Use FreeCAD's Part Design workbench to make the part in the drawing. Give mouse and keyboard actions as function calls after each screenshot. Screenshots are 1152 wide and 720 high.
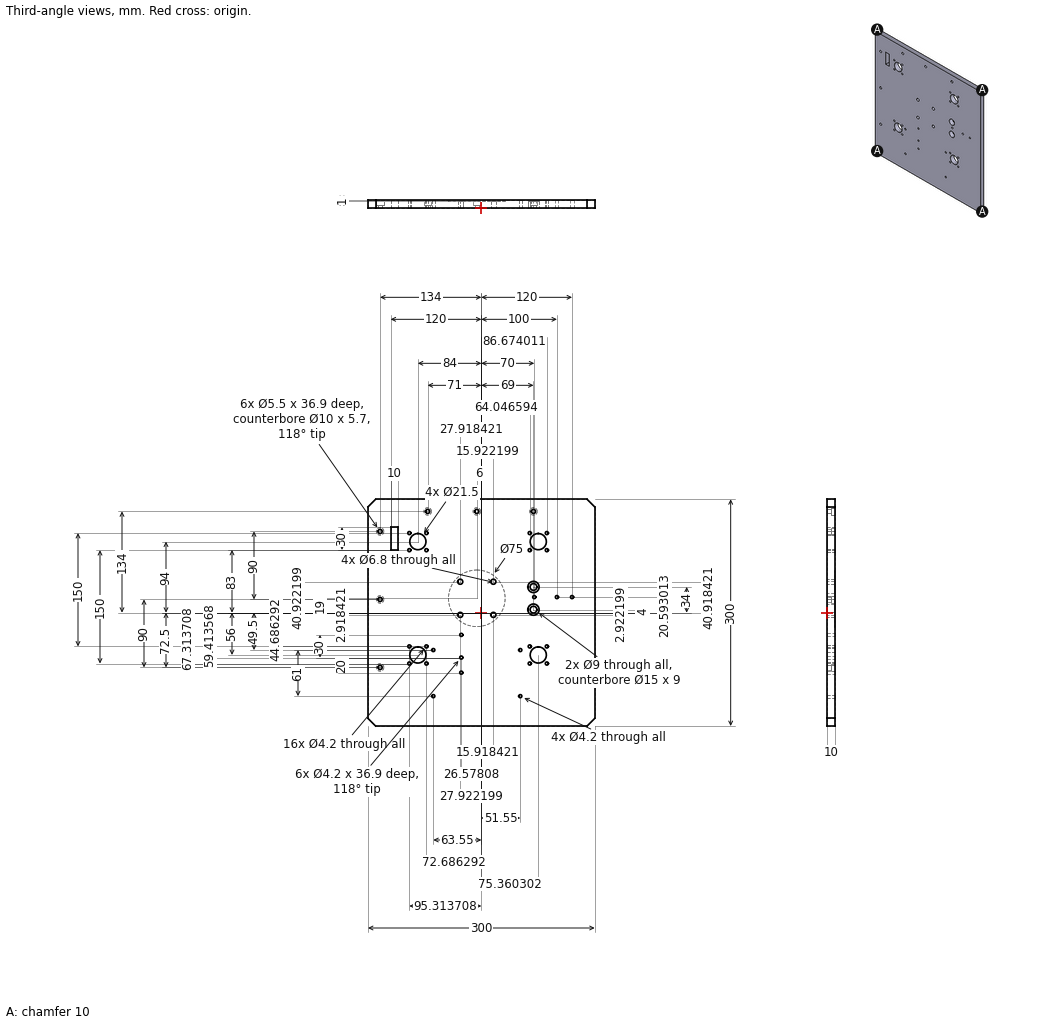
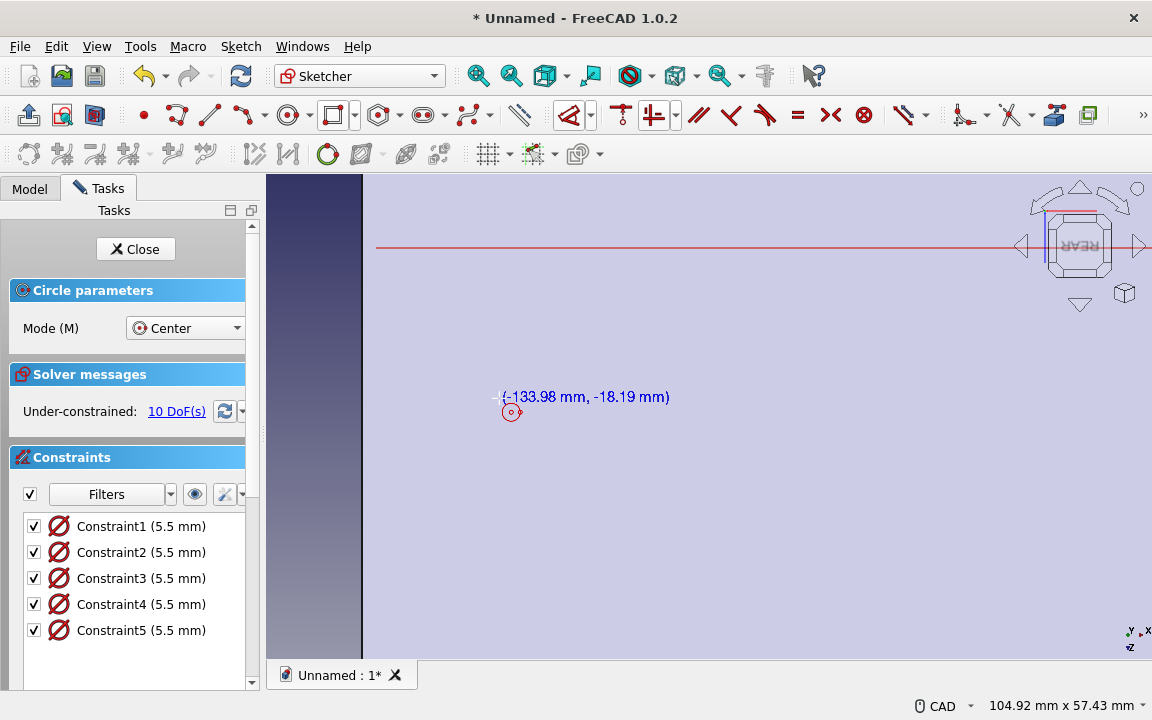
scroll(499, 398, down, 9)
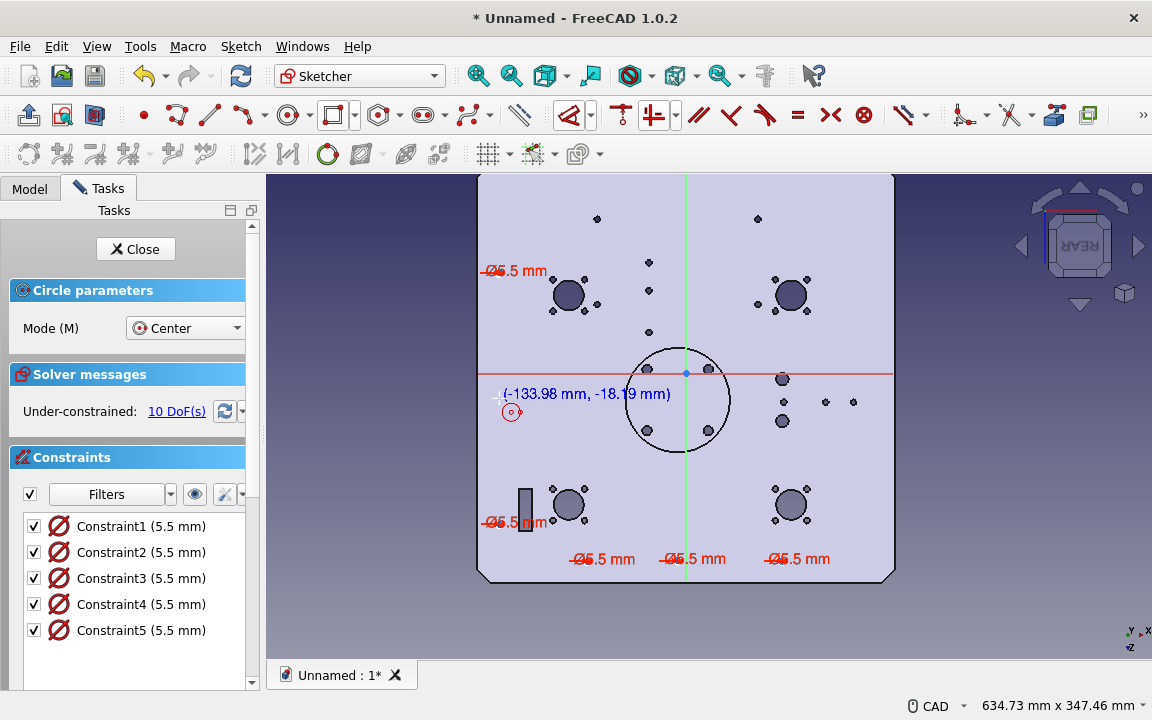
click(499, 398)
move(502, 395)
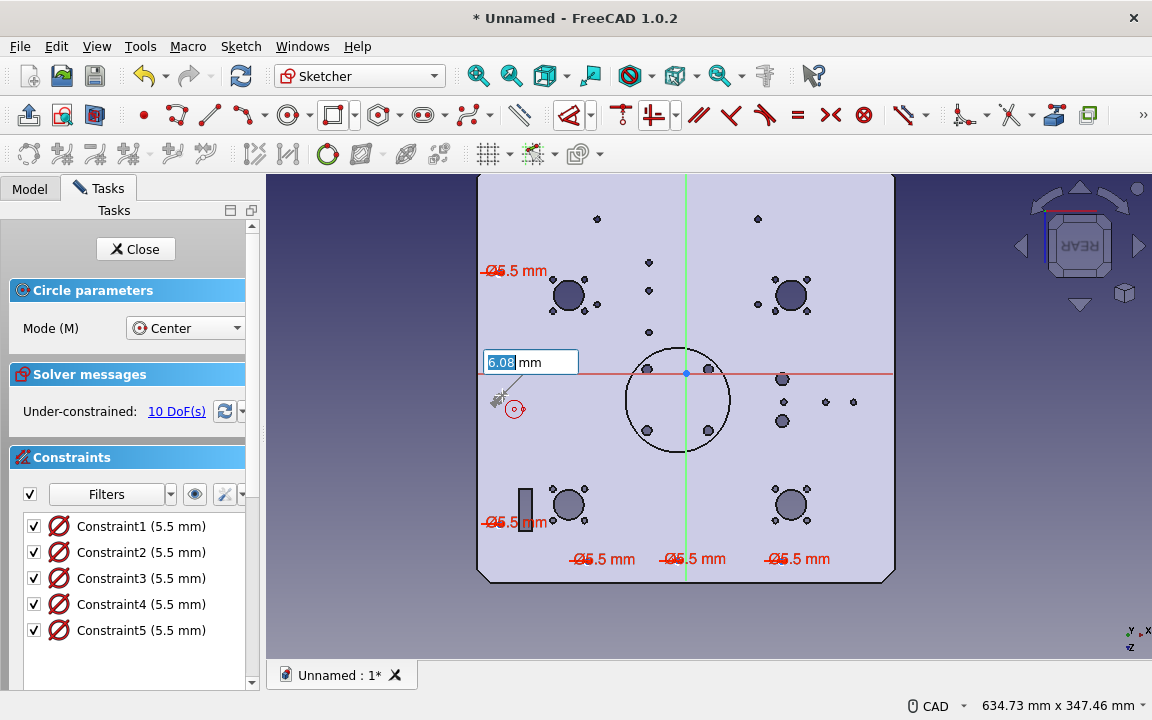
text(5.5)
key(Return)
key(Escape)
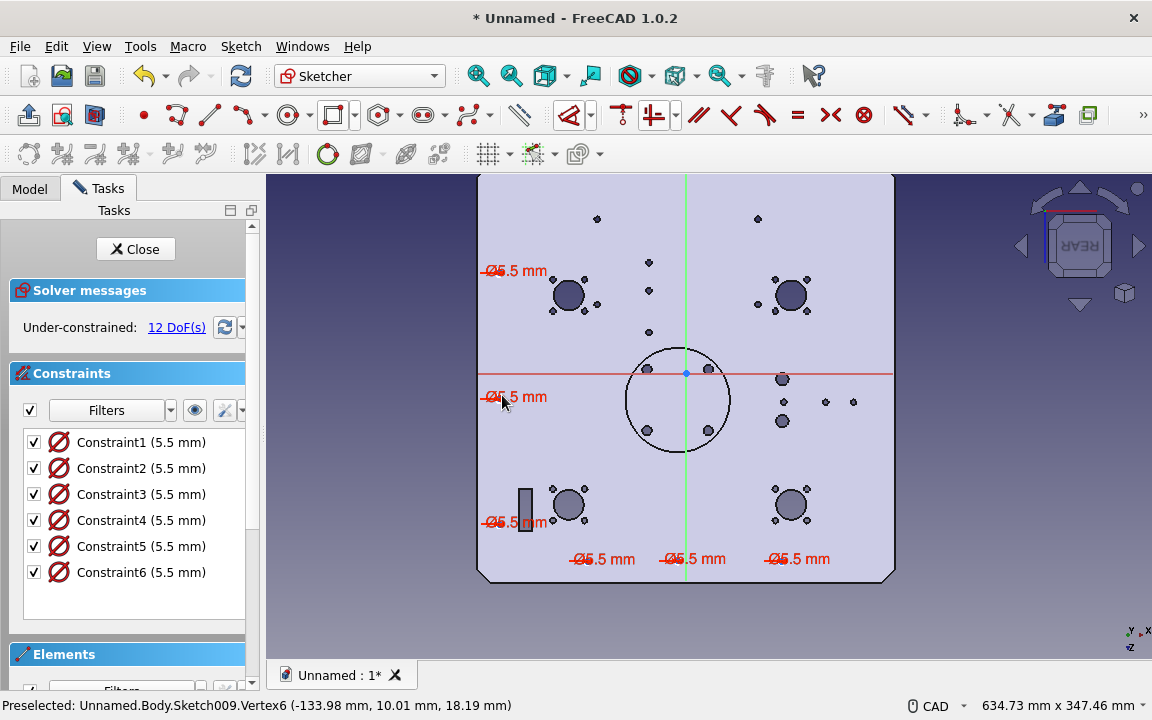
click(587, 561)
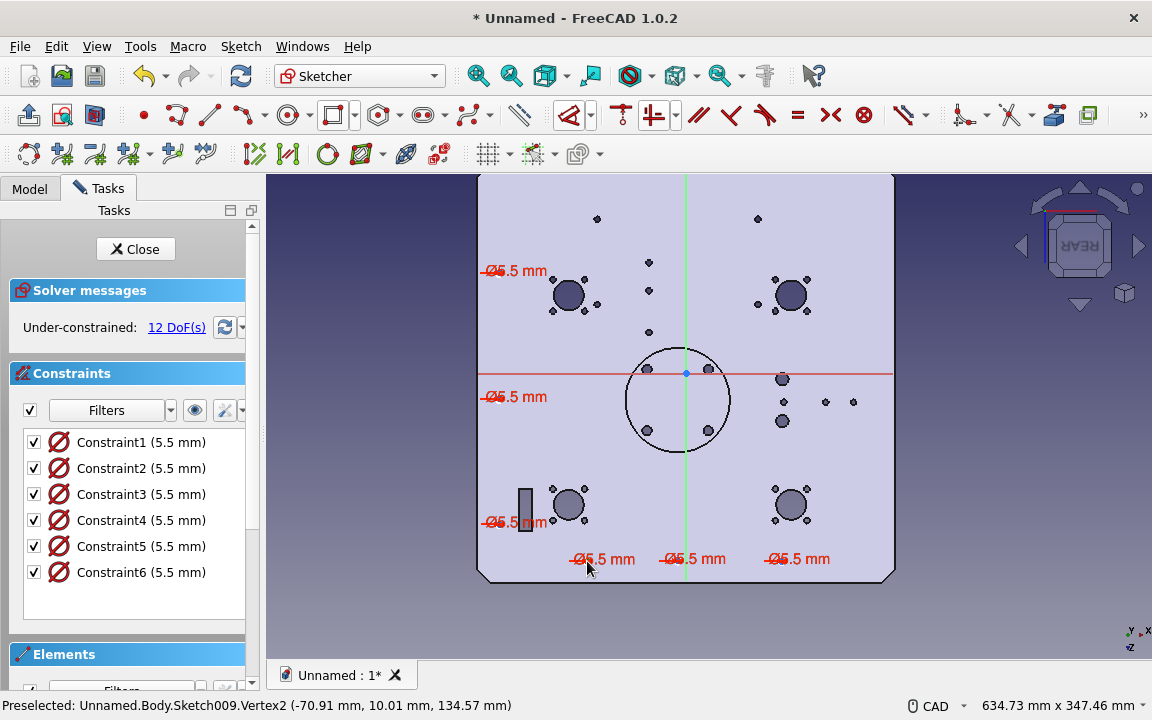
click(678, 561)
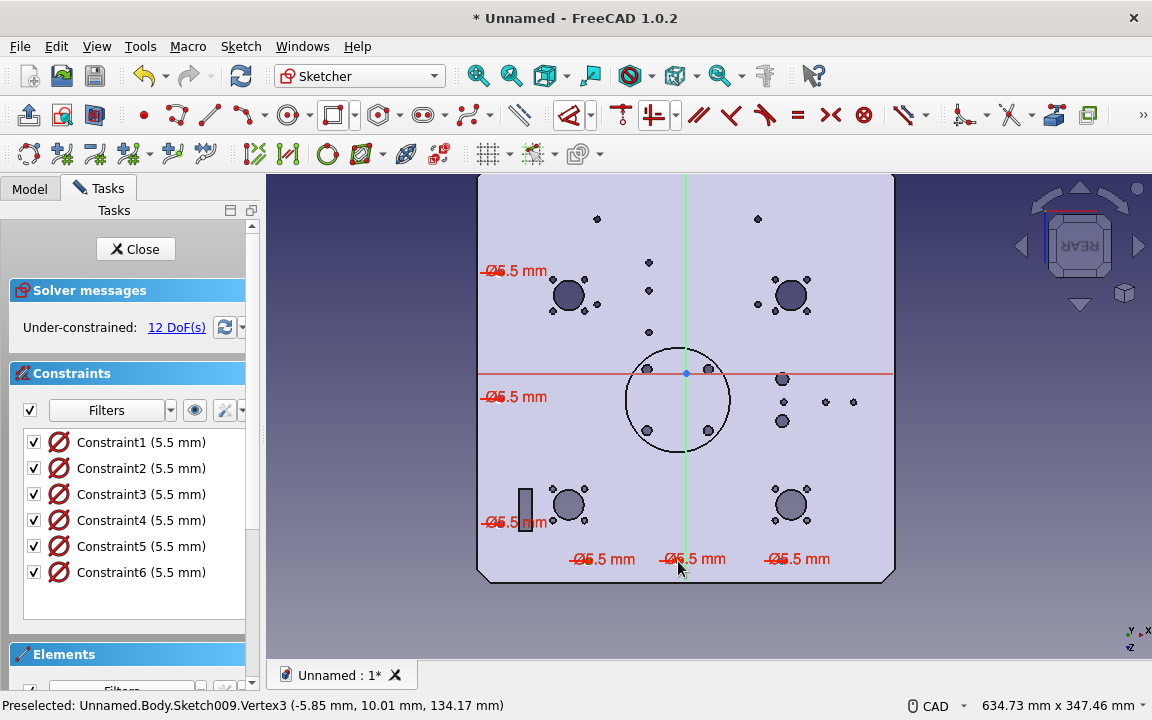
click(676, 116)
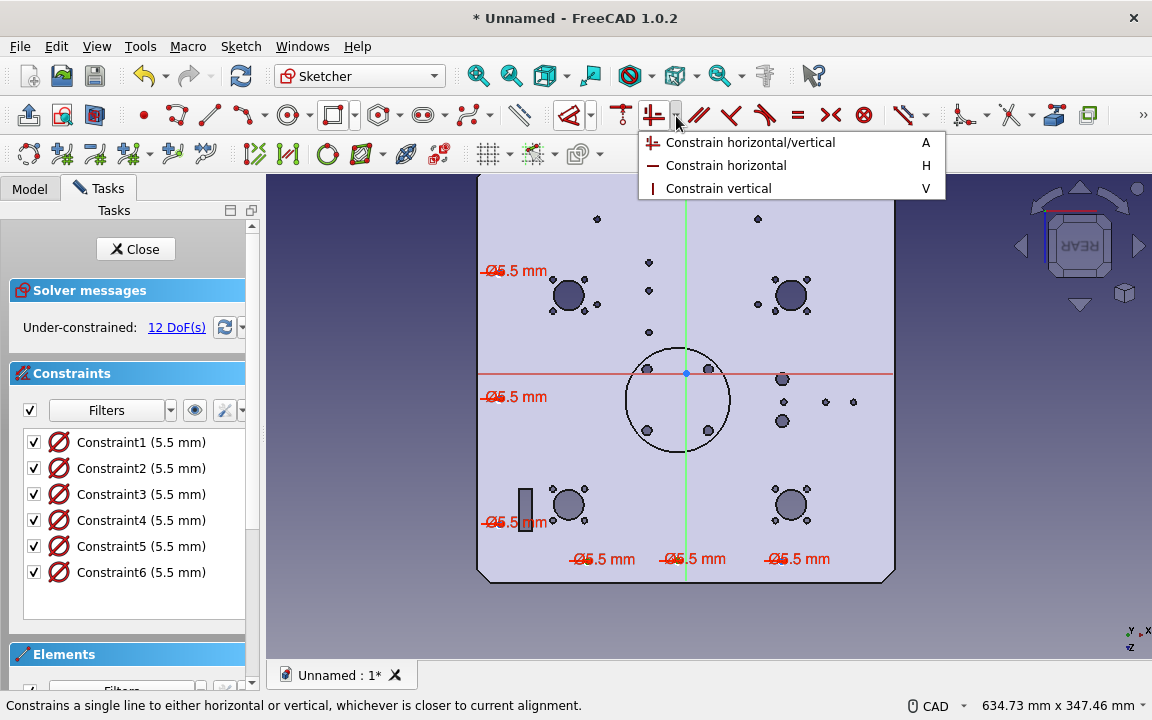
click(792, 166)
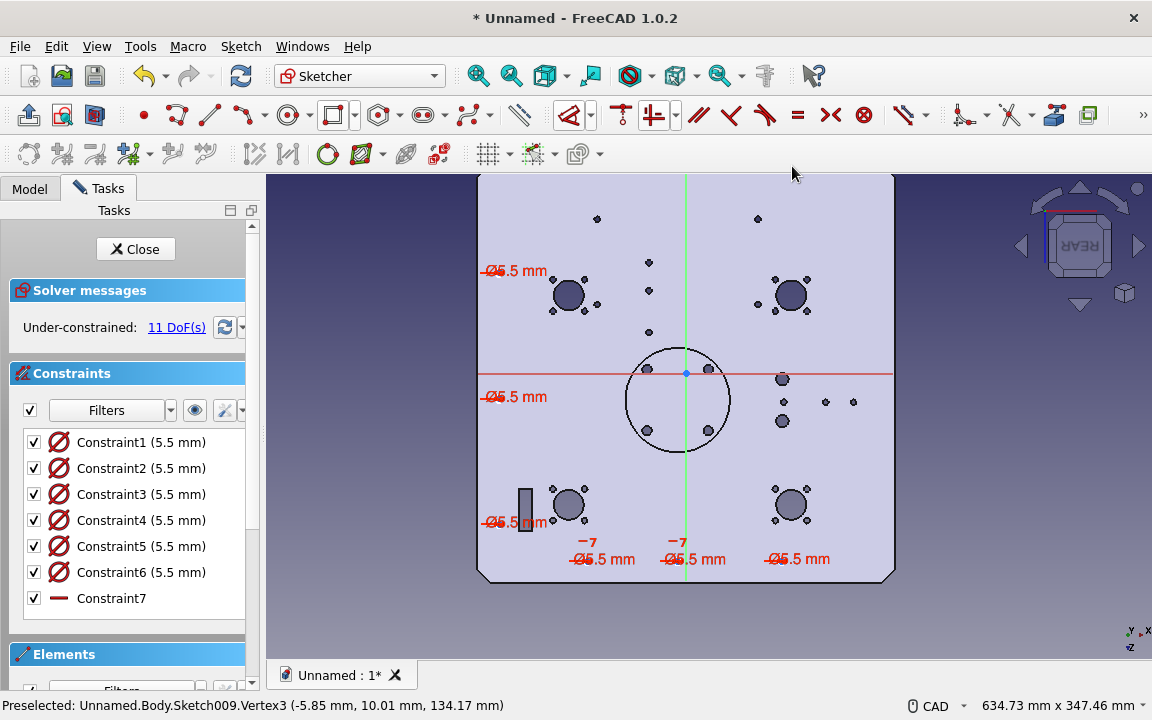
click(678, 561)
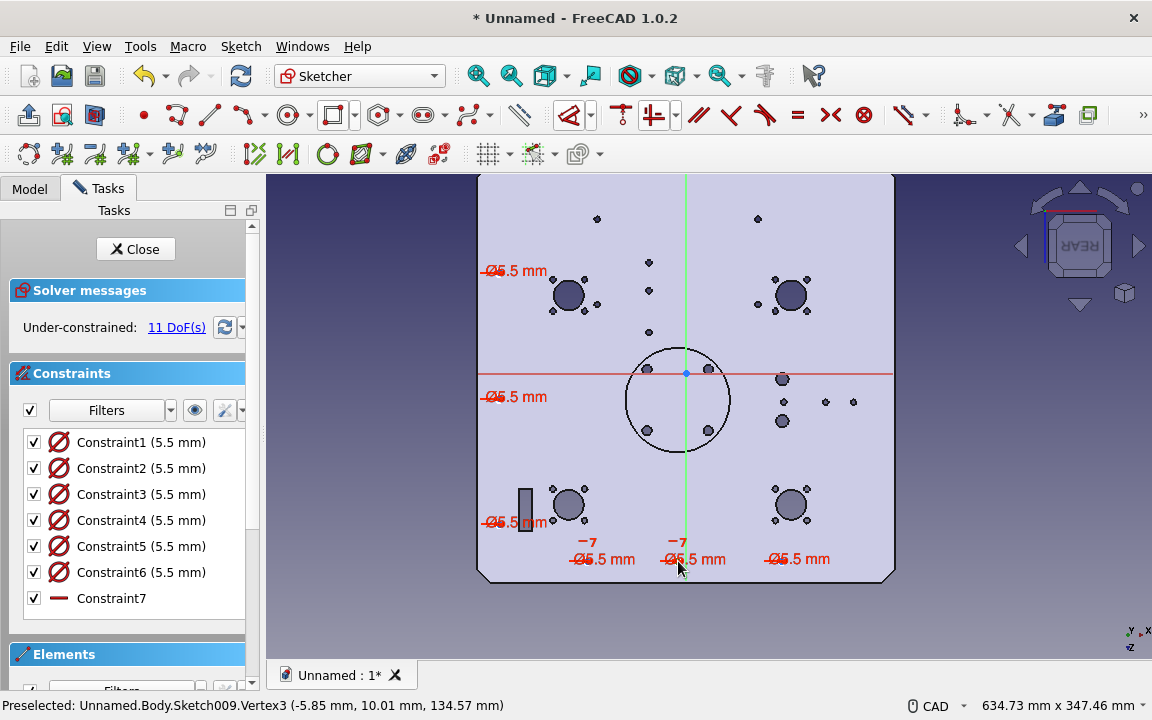
click(782, 561)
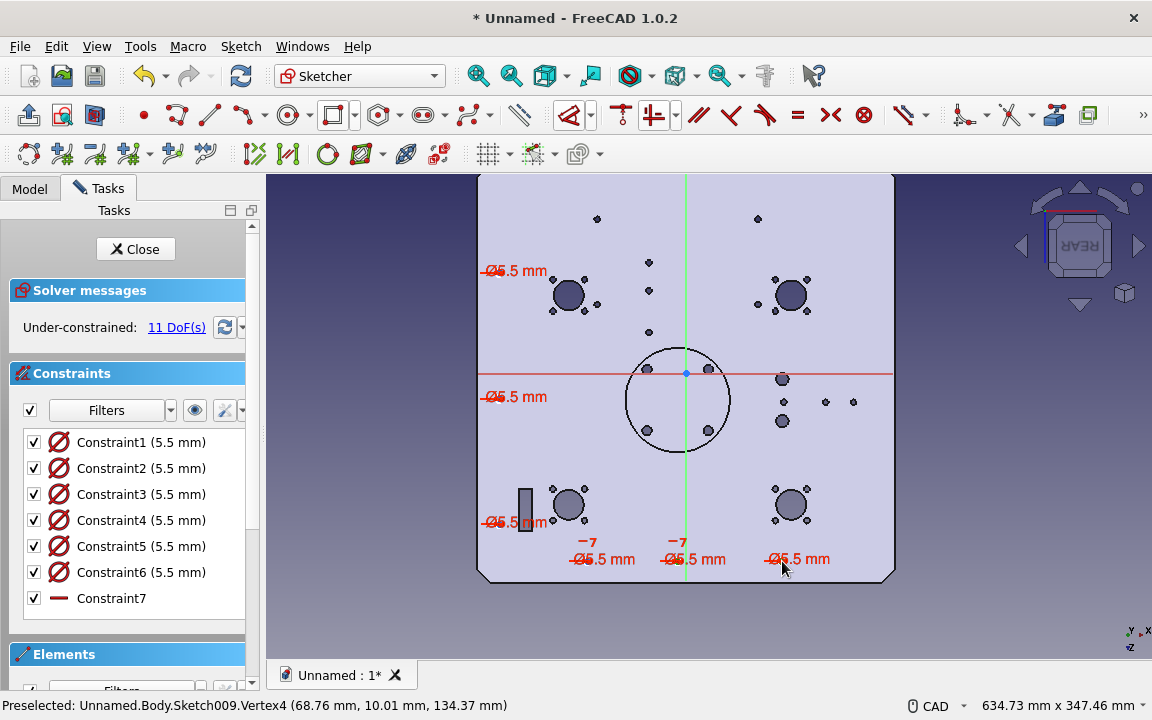
click(676, 116)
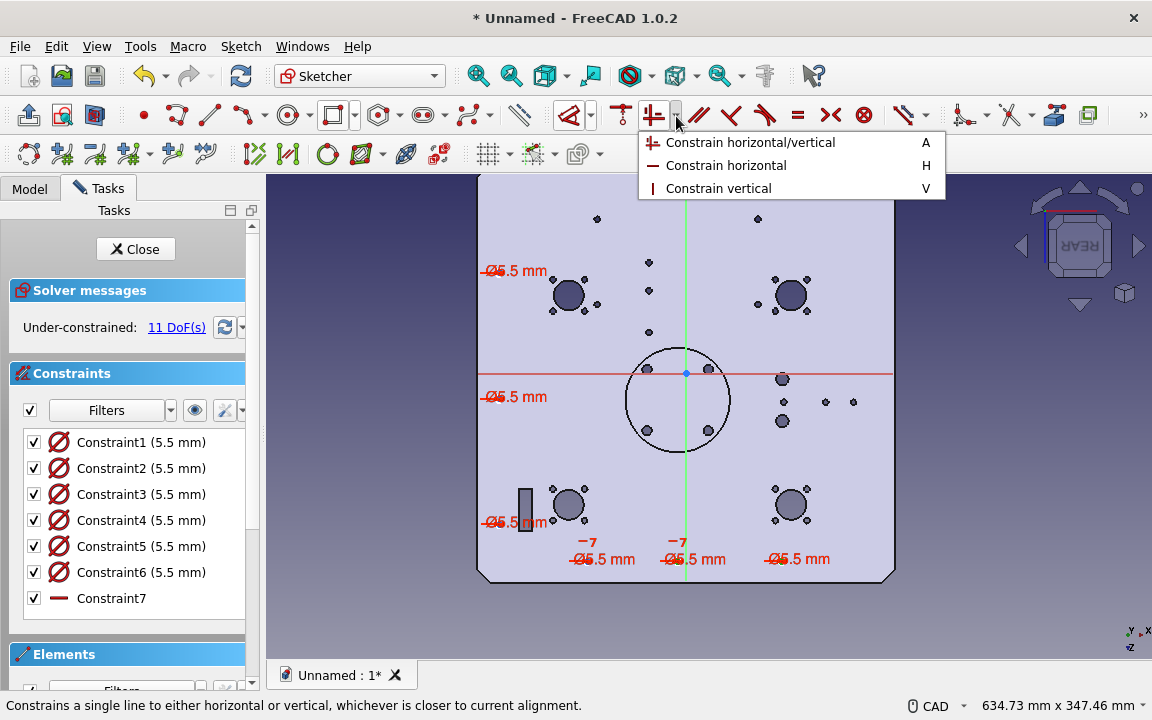
click(792, 166)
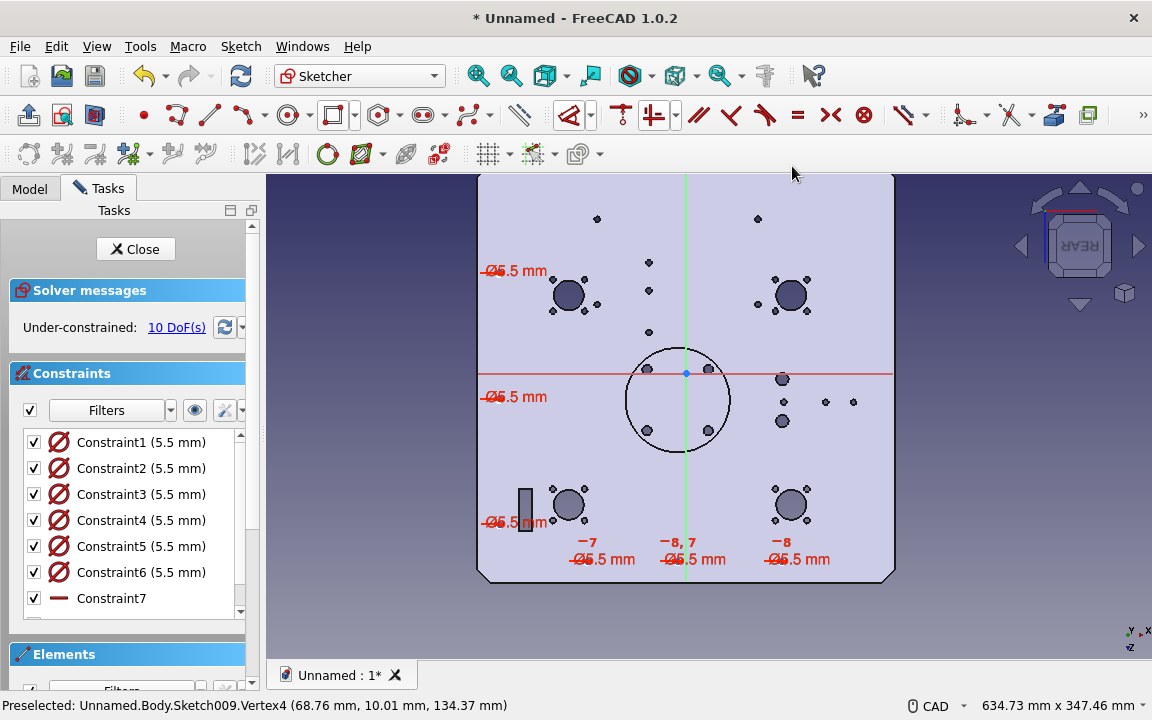
click(499, 524)